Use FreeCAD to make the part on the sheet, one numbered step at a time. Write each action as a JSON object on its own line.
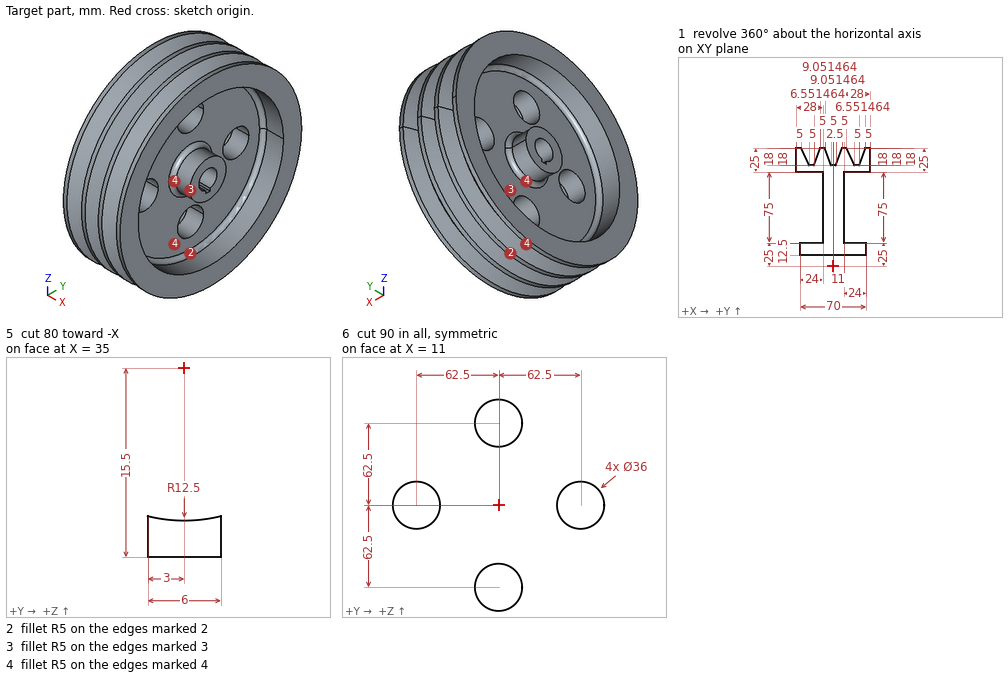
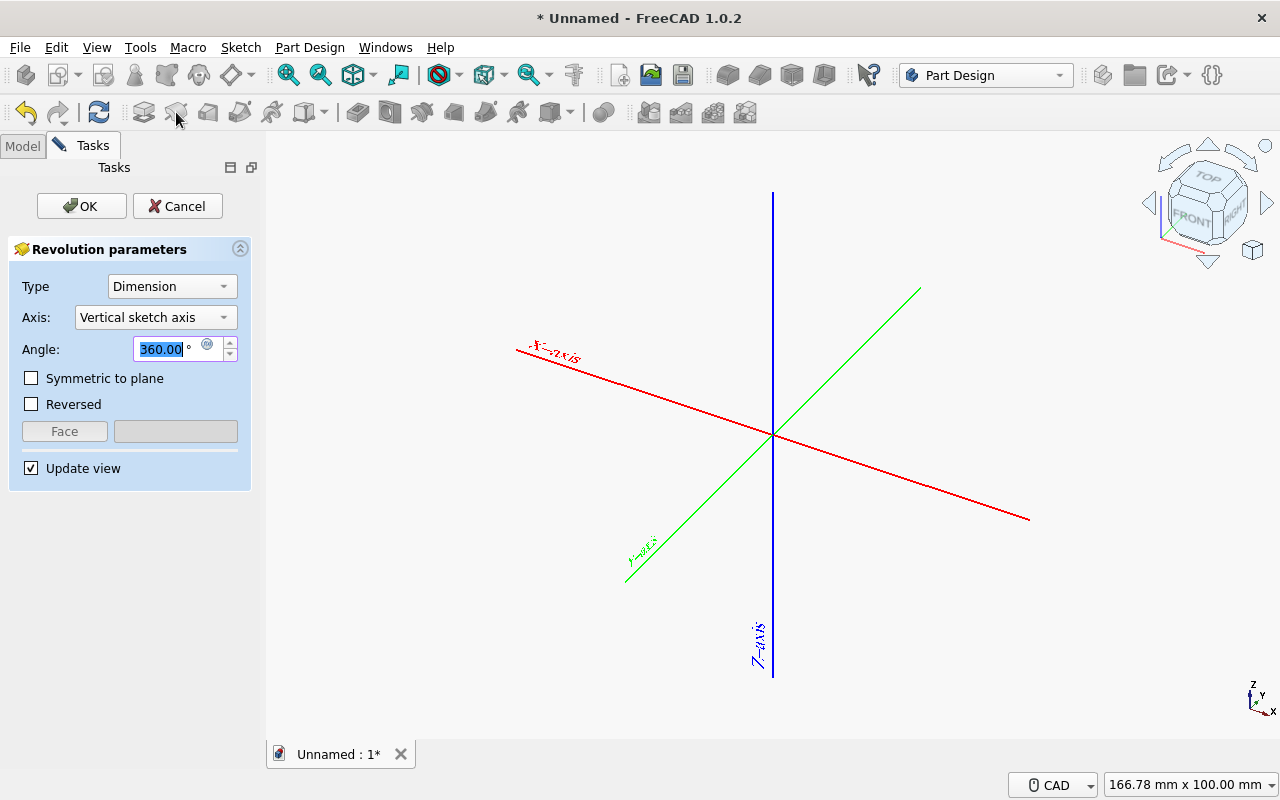
{"action": "left_click", "coordinate": [156, 318]}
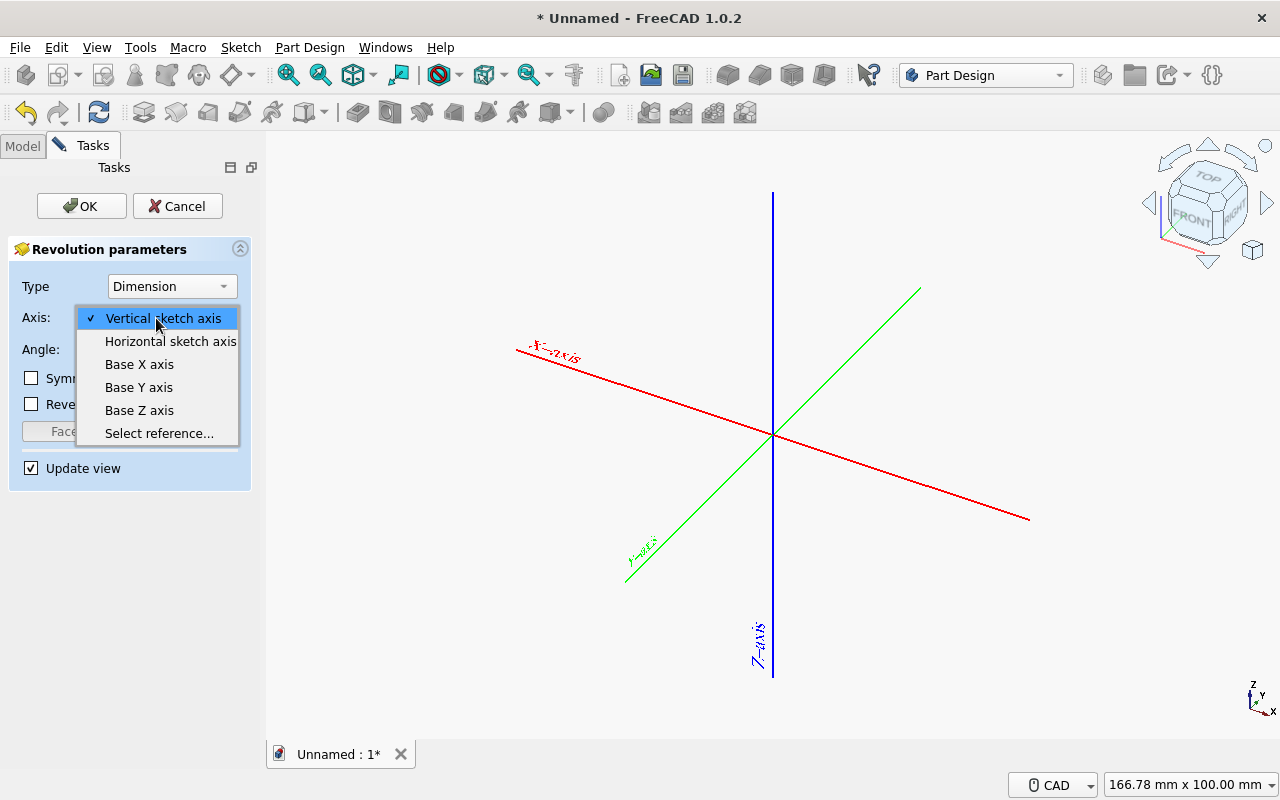
{"action": "left_click", "coordinate": [156, 342]}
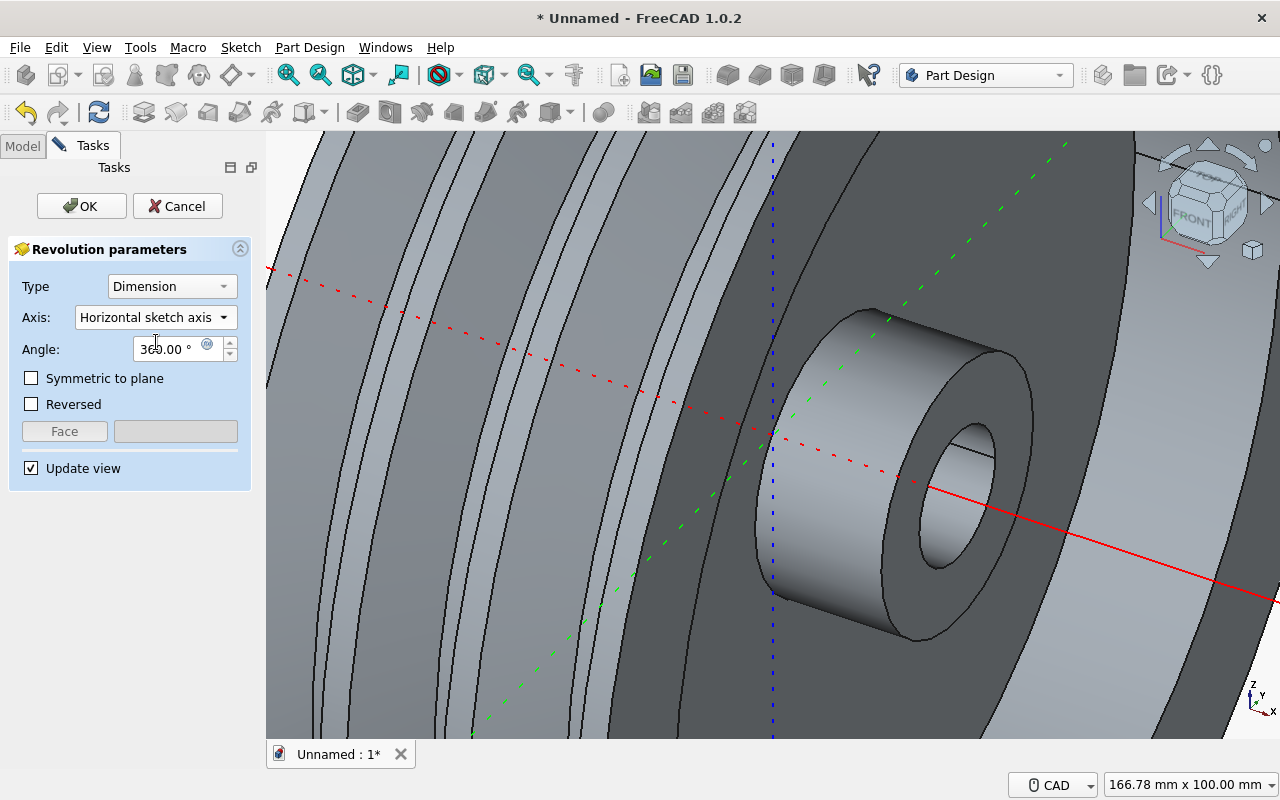
{"action": "left_click", "coordinate": [82, 206]}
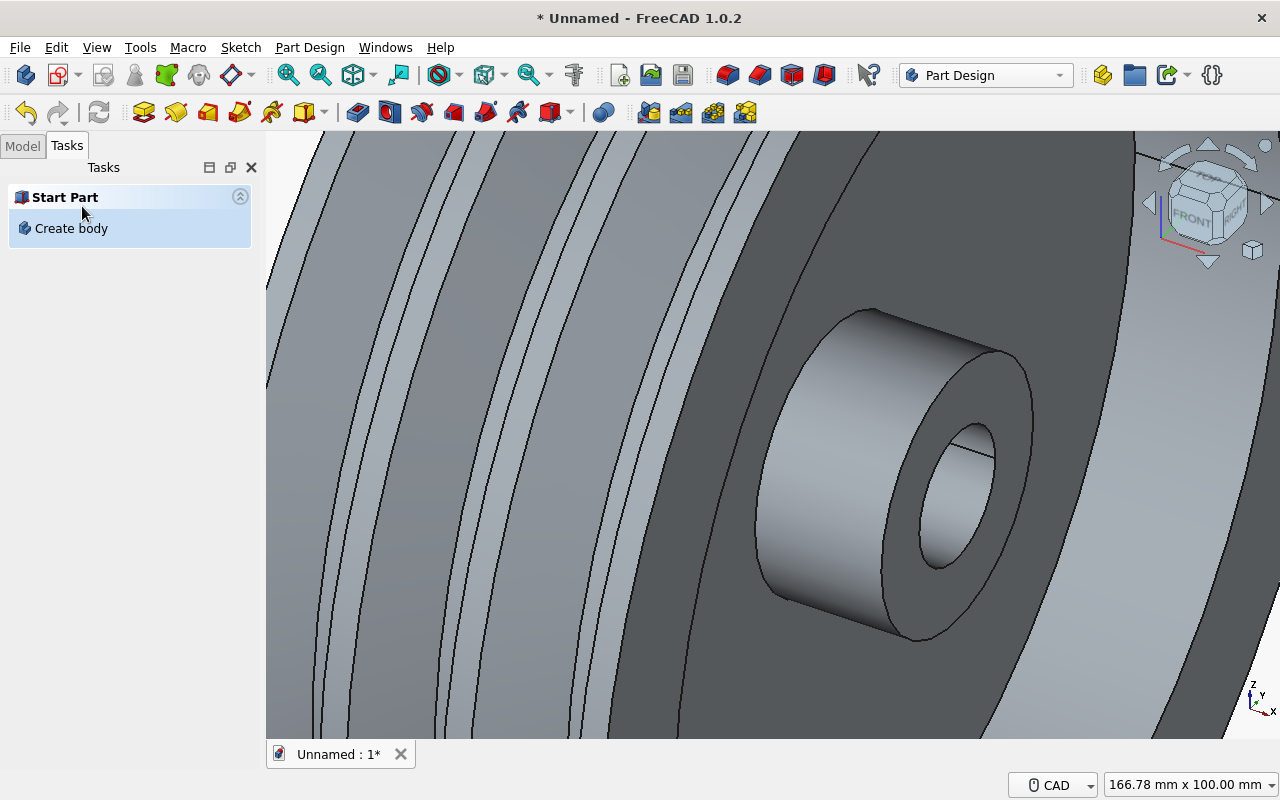
{"action": "left_click", "coordinate": [290, 76]}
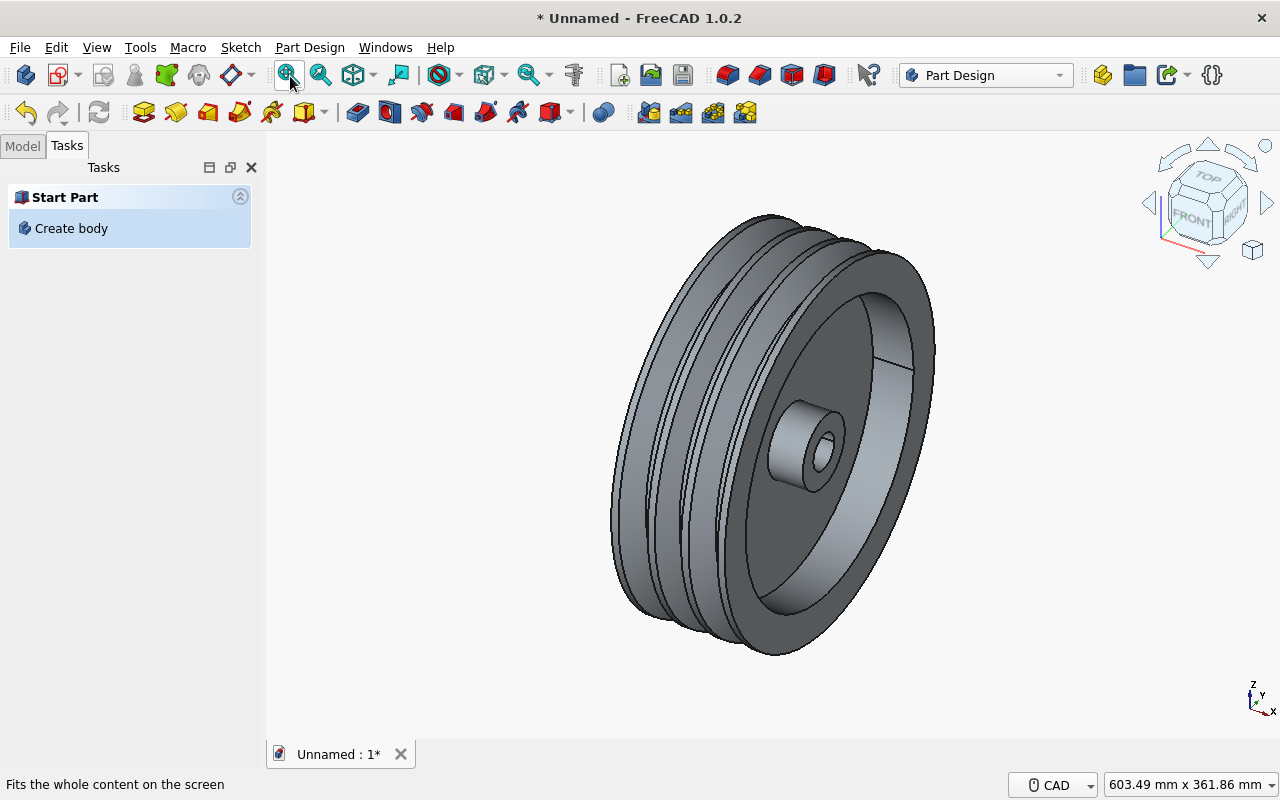
{"action": "key", "text": "0"}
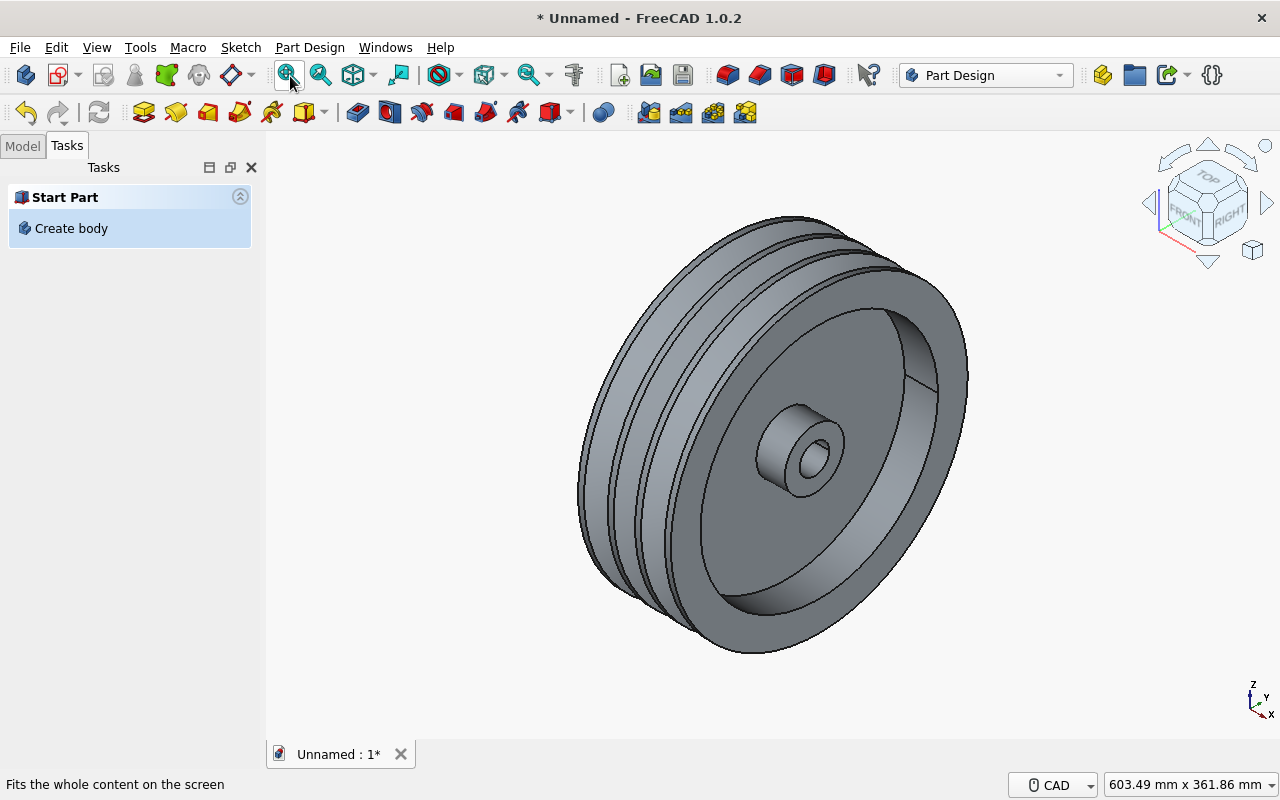
{"action": "key", "text": "2"}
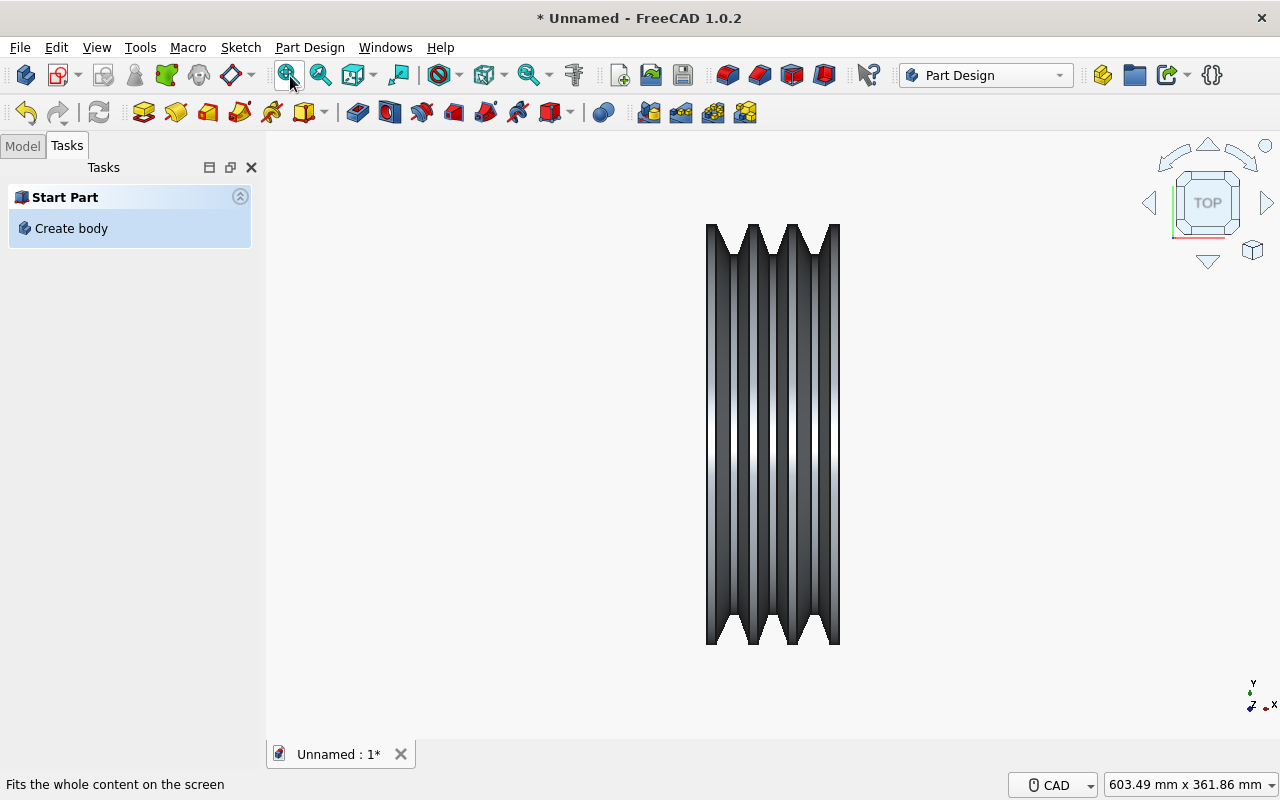
{"action": "key", "text": "1"}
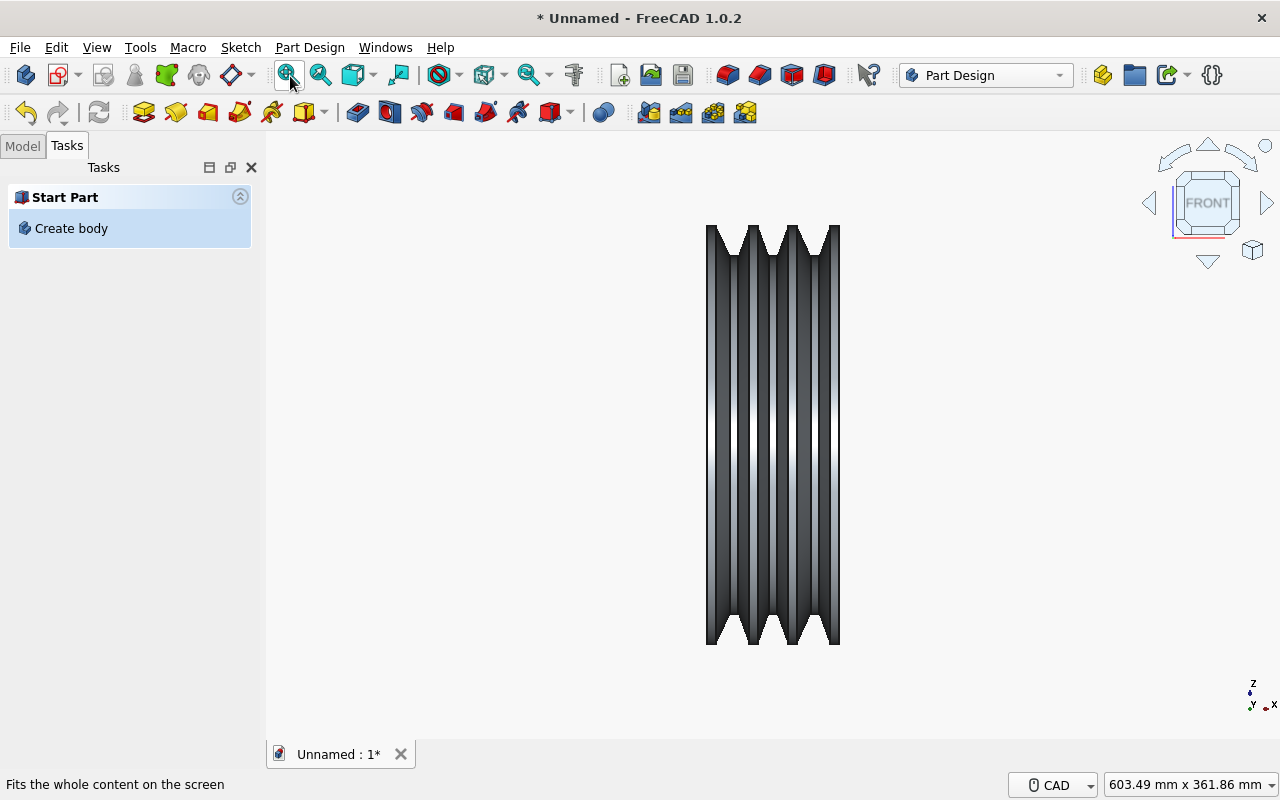
{"action": "key", "text": "3"}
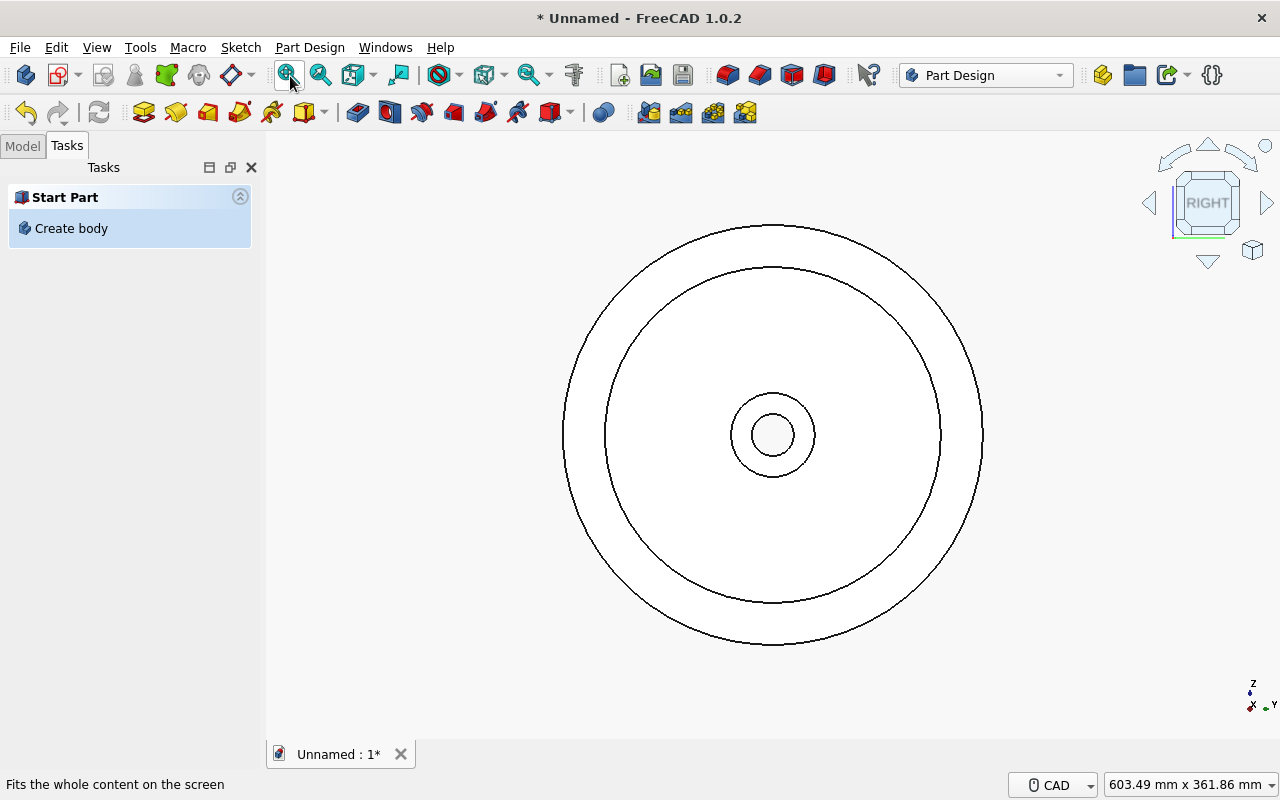
{"action": "key", "text": "5"}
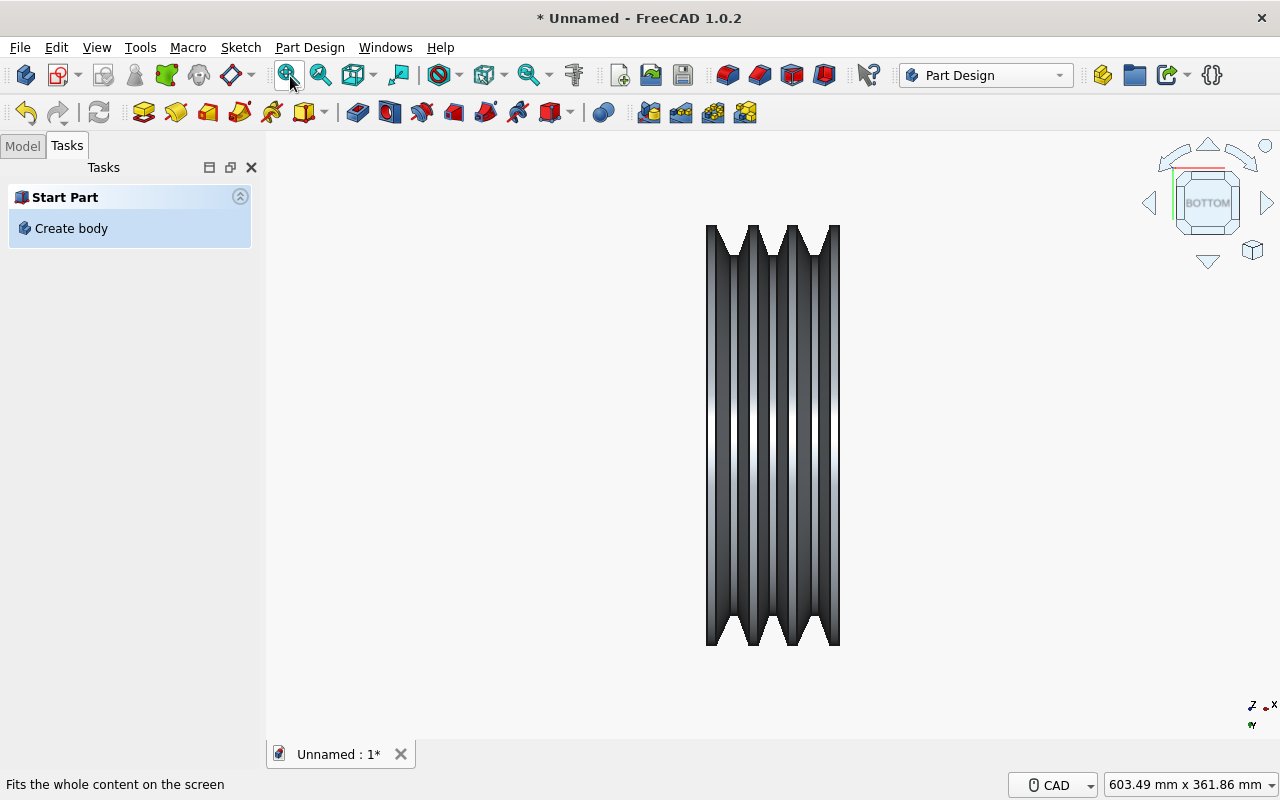
{"action": "key", "text": "4"}